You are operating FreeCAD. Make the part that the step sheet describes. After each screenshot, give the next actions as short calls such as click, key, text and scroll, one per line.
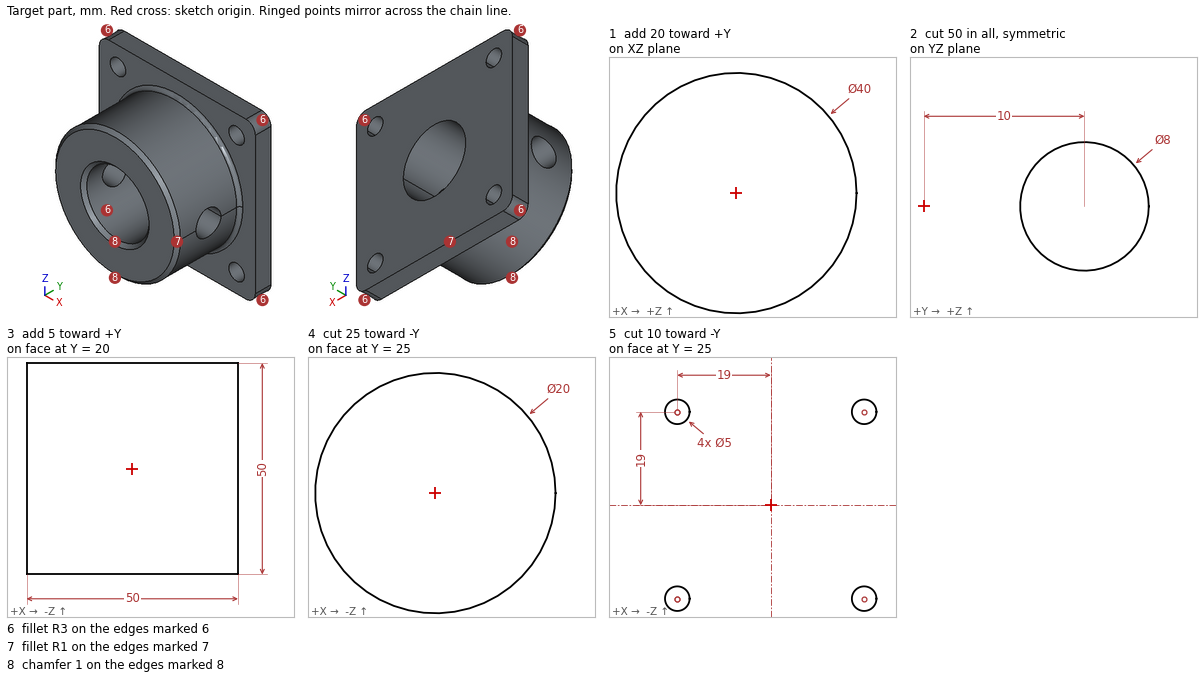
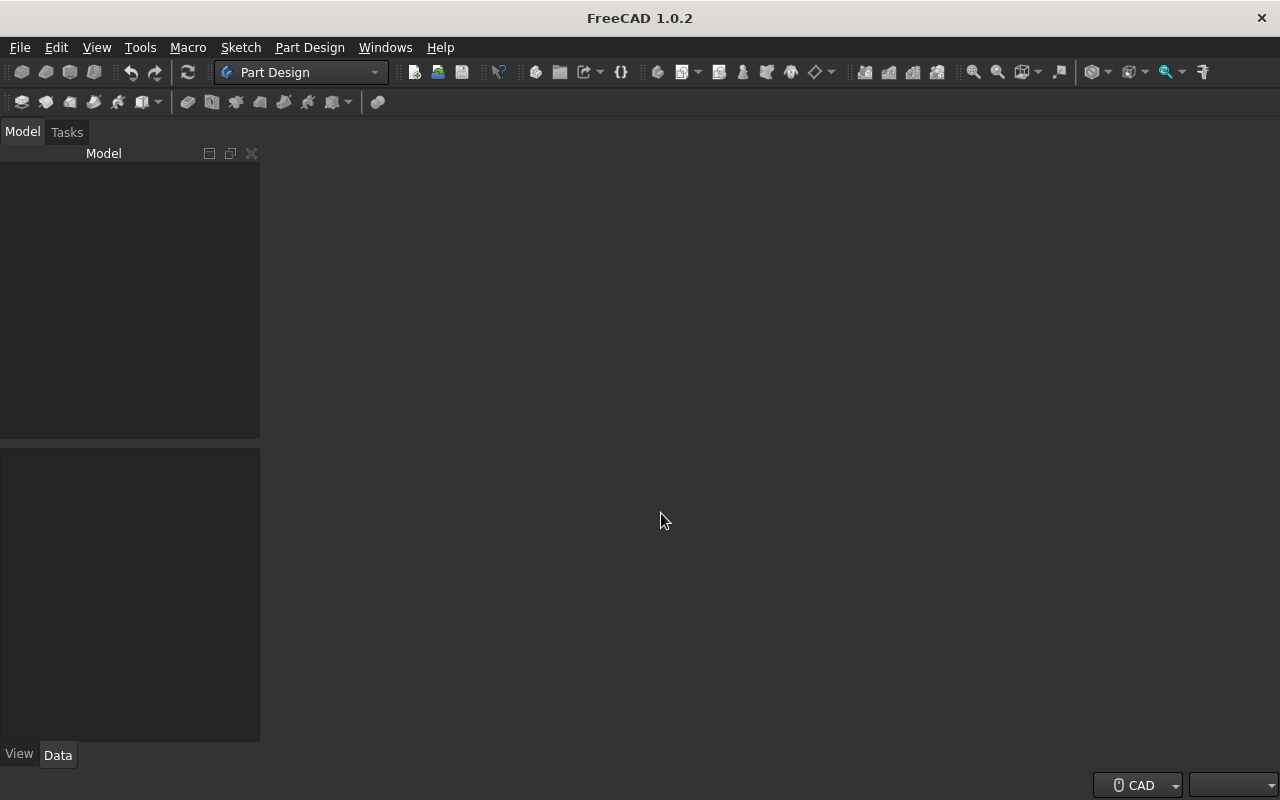
click(414, 72)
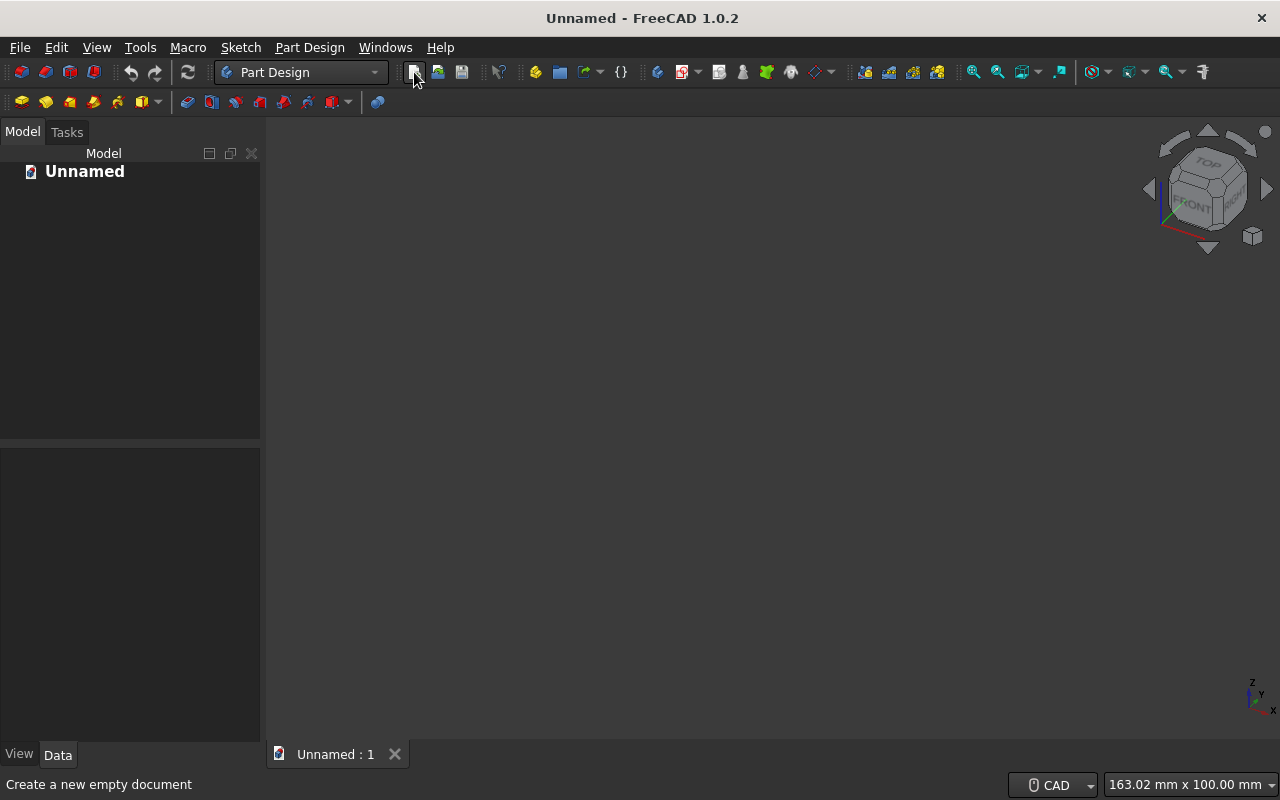
click(682, 72)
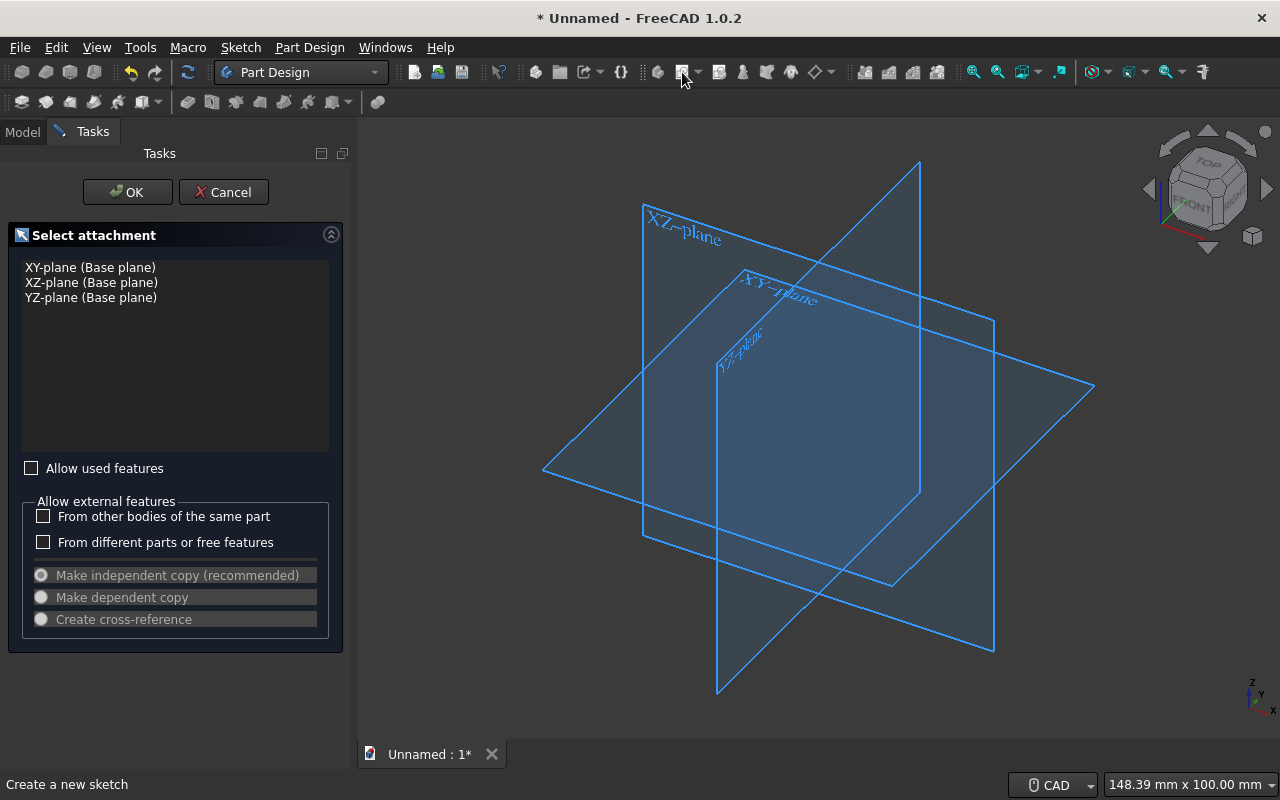
click(82, 282)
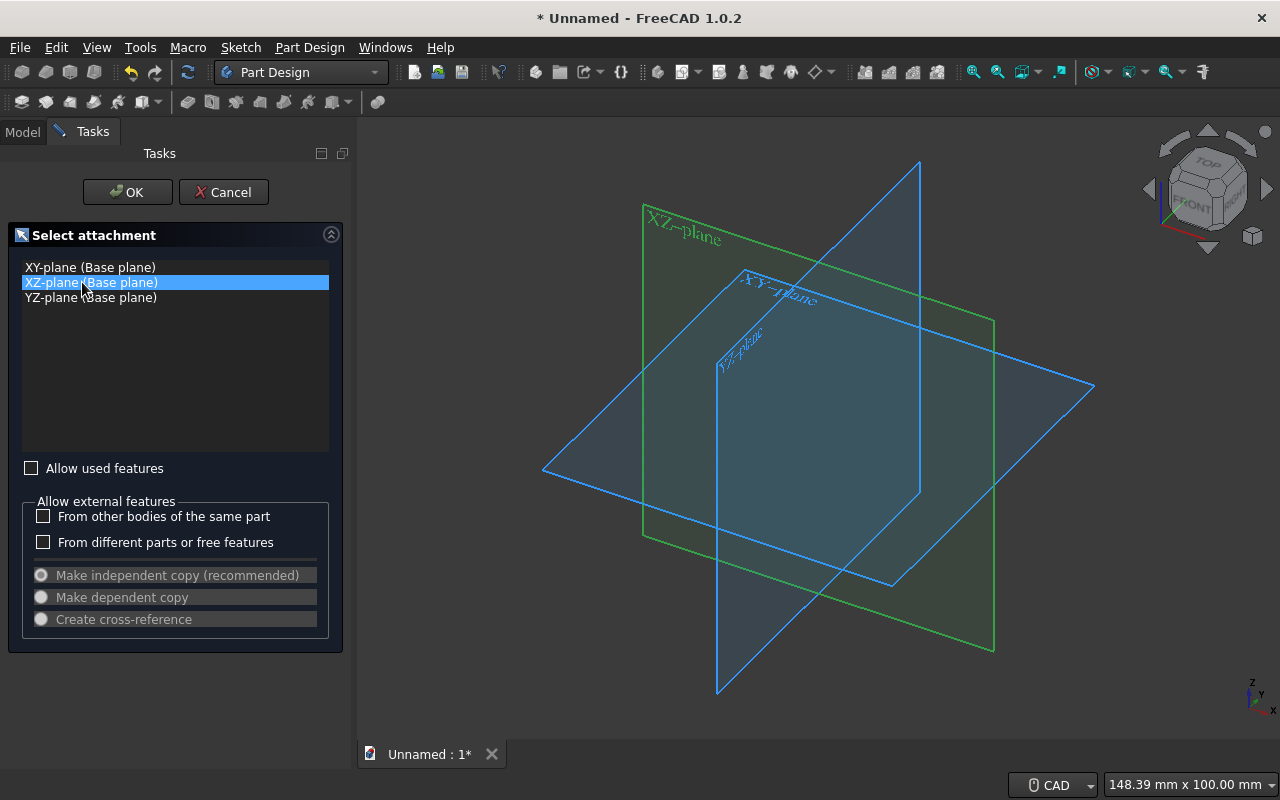
click(128, 192)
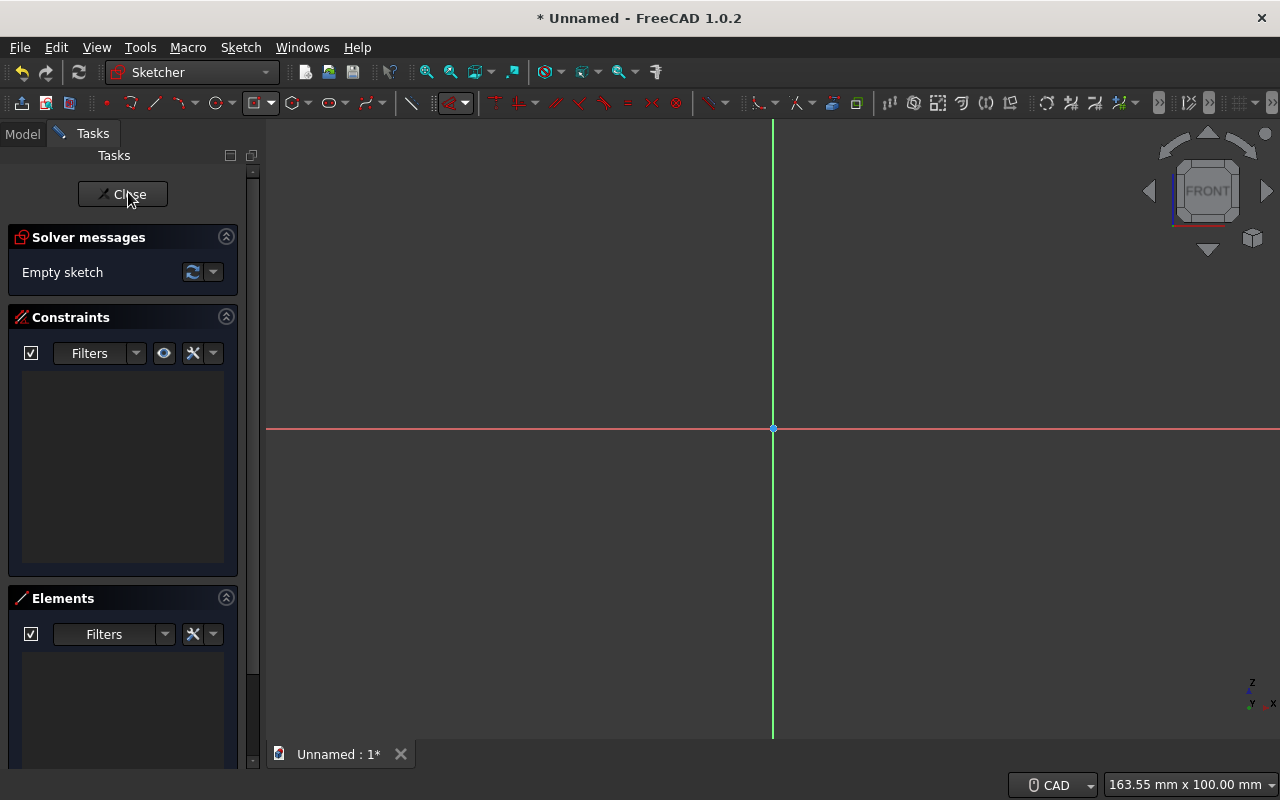
scroll(912, 429, up, 2)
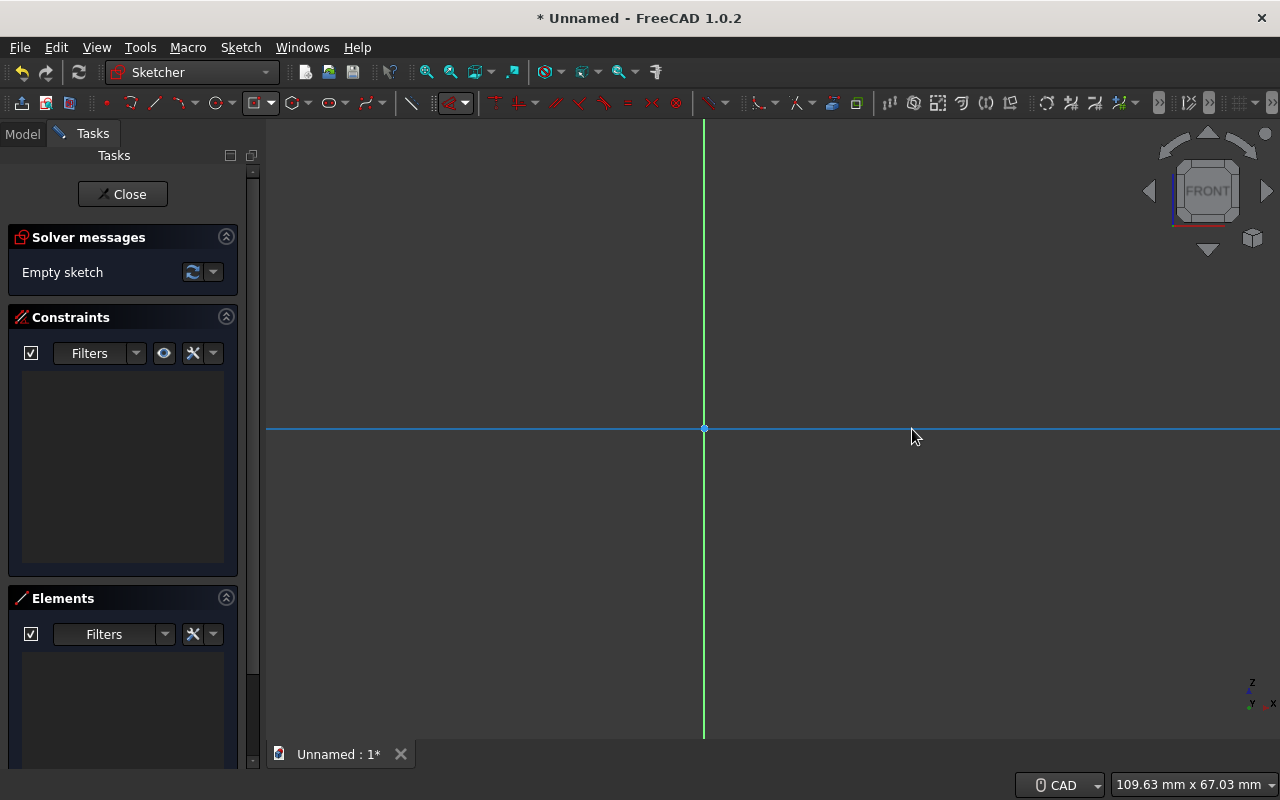
click(216, 104)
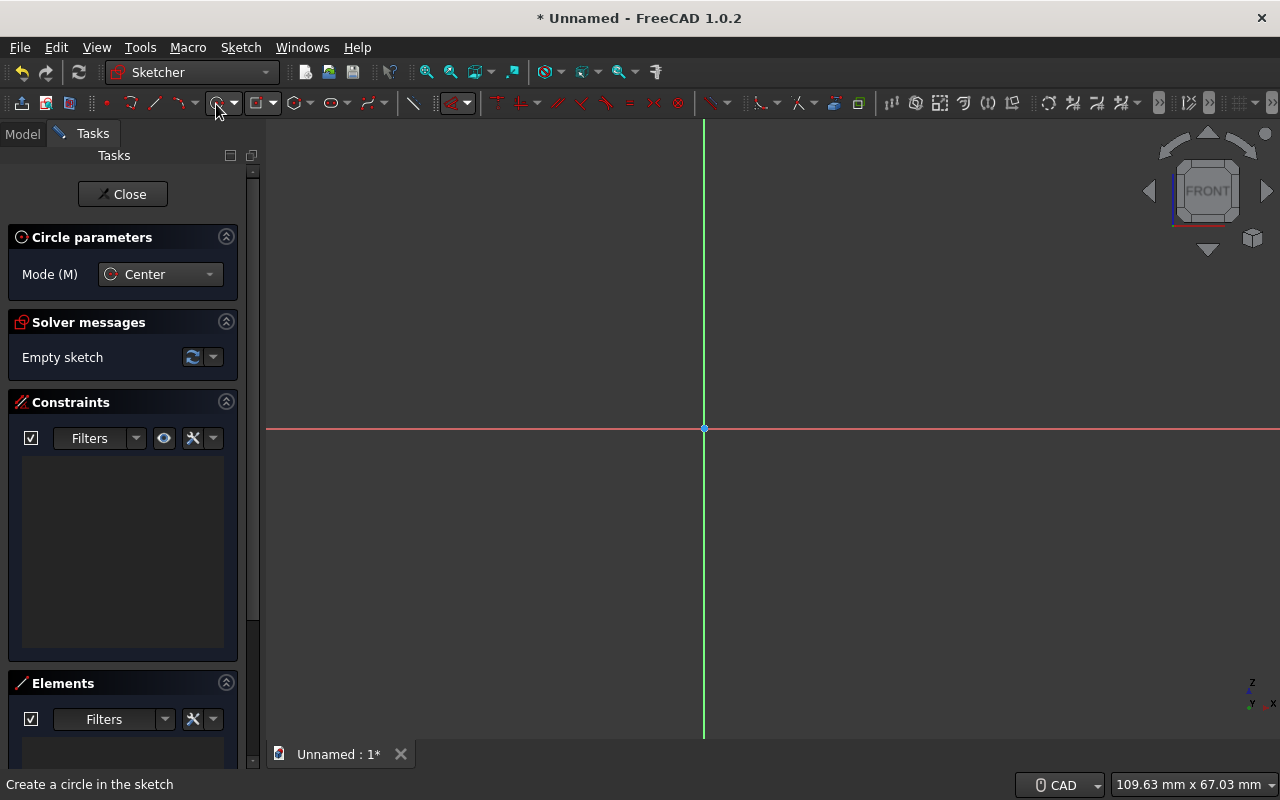
click(704, 429)
click(835, 298)
key(Escape)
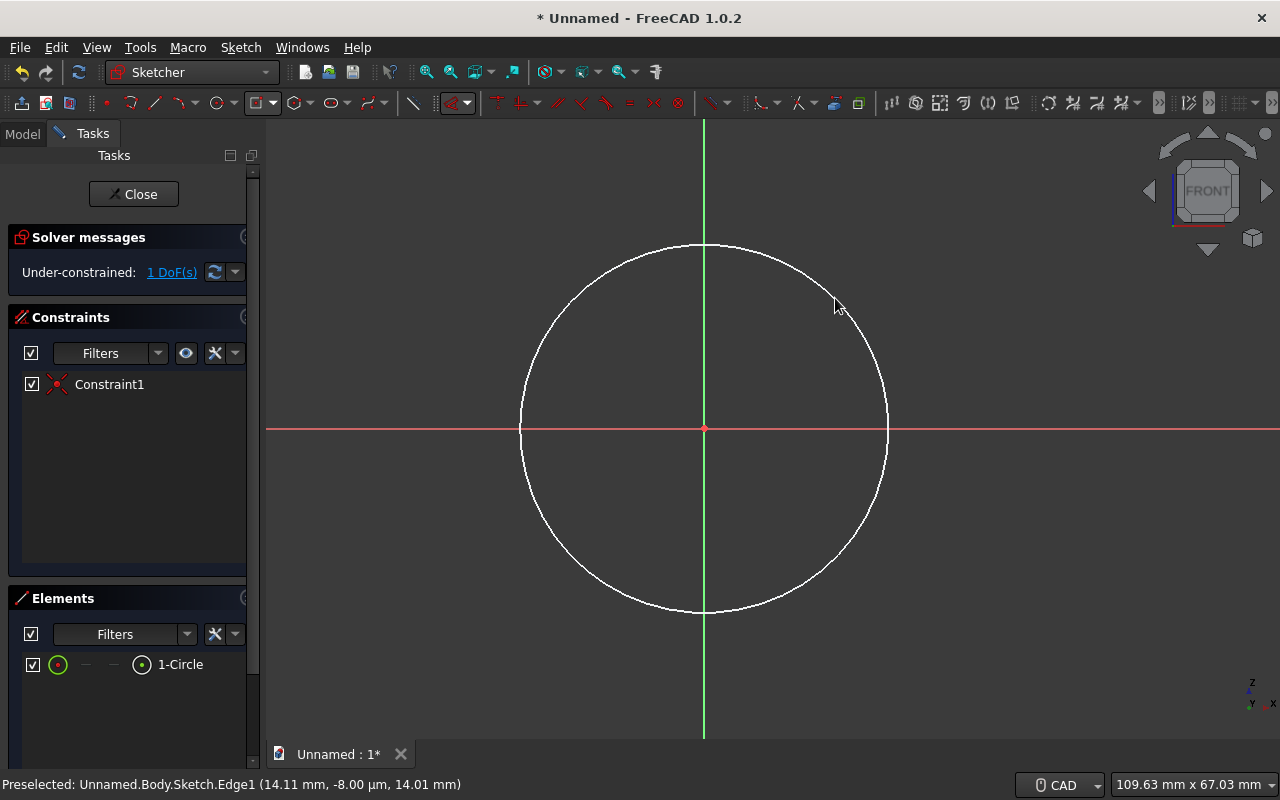
click(834, 298)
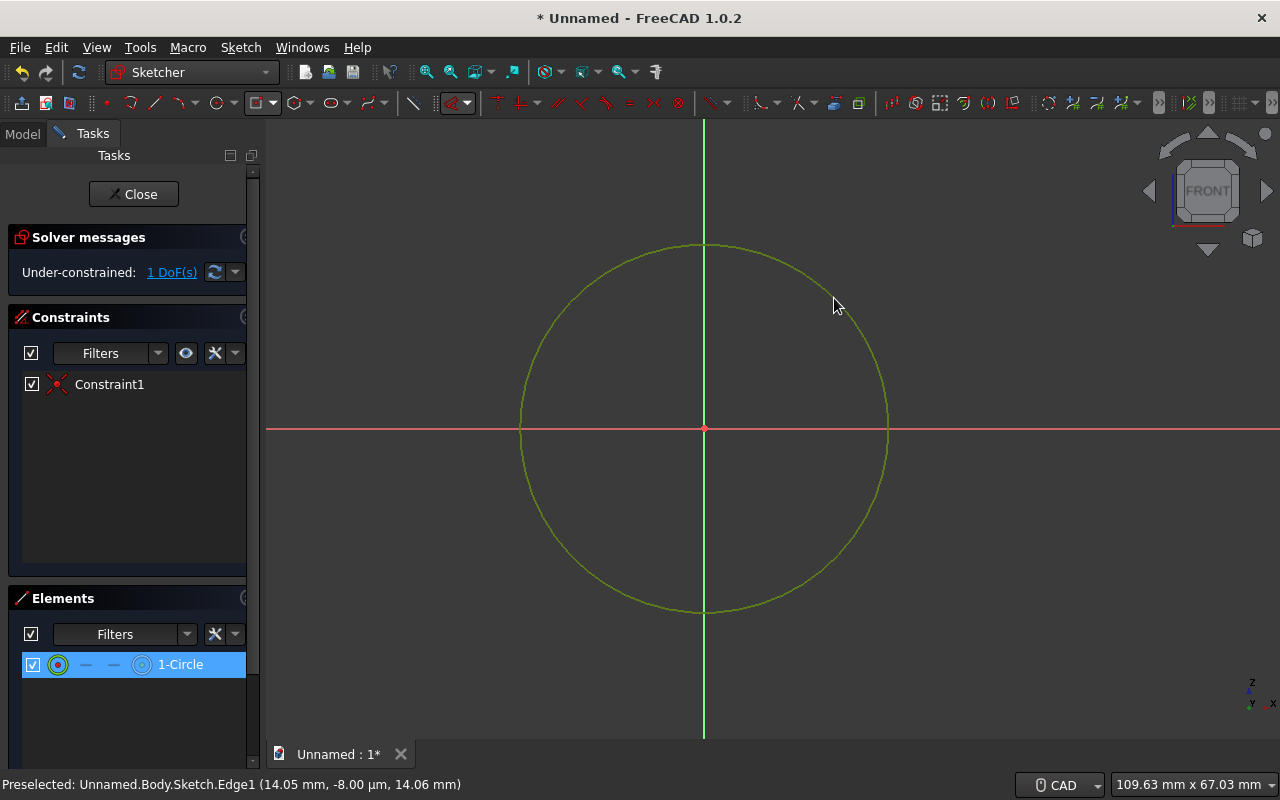
click(470, 104)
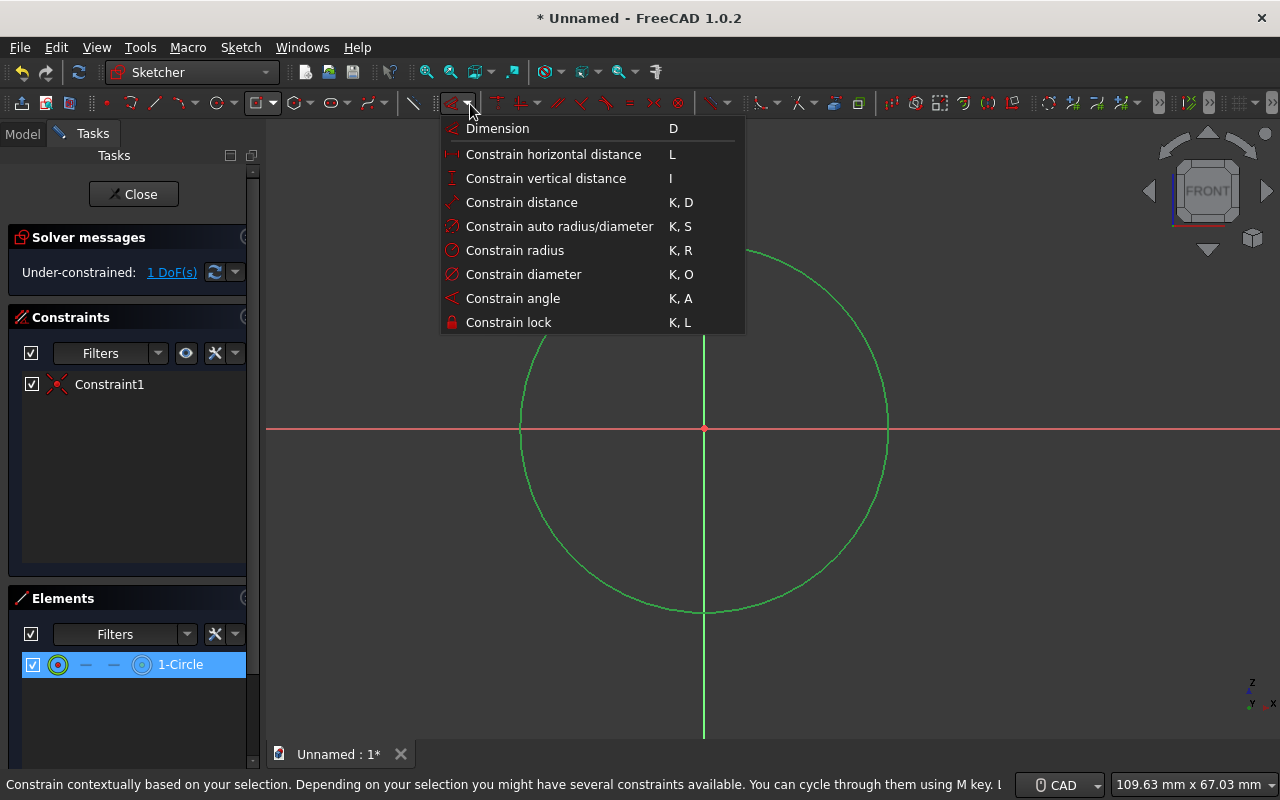
click(593, 274)